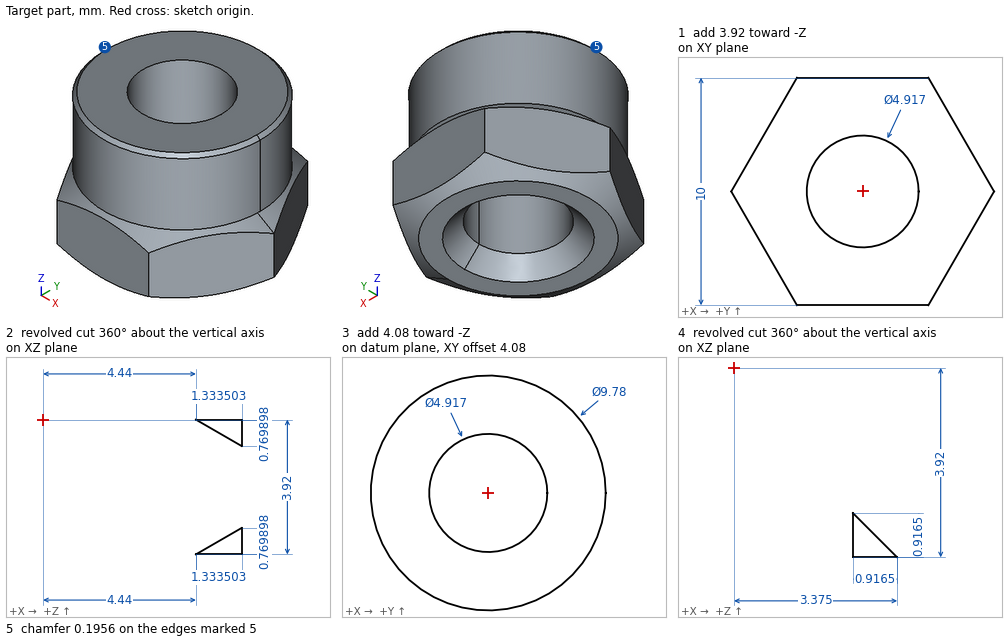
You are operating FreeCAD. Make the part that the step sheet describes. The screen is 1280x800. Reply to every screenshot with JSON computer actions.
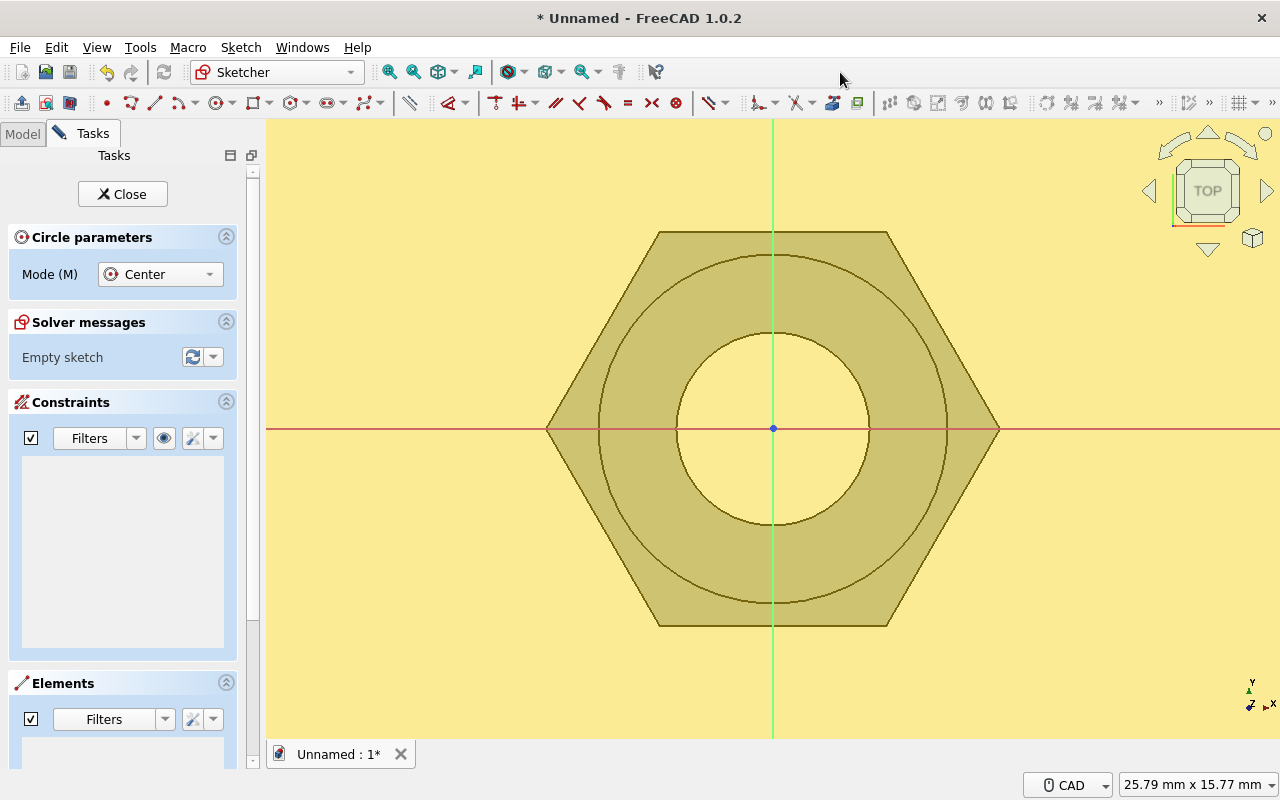
{"action": "left_click", "coordinate": [773, 429]}
{"action": "mouse_move", "coordinate": [909, 293]}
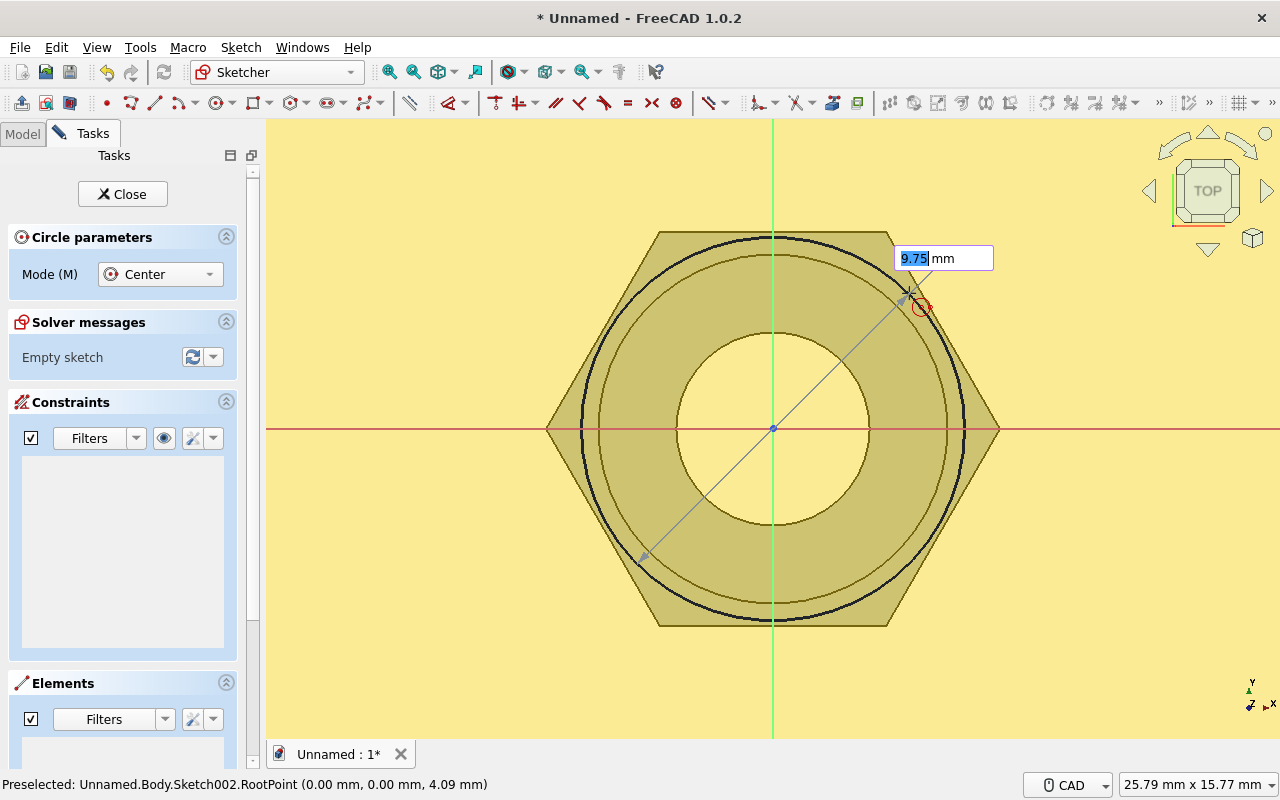
{"action": "type", "text": "9.78"}
{"action": "key", "text": "Return"}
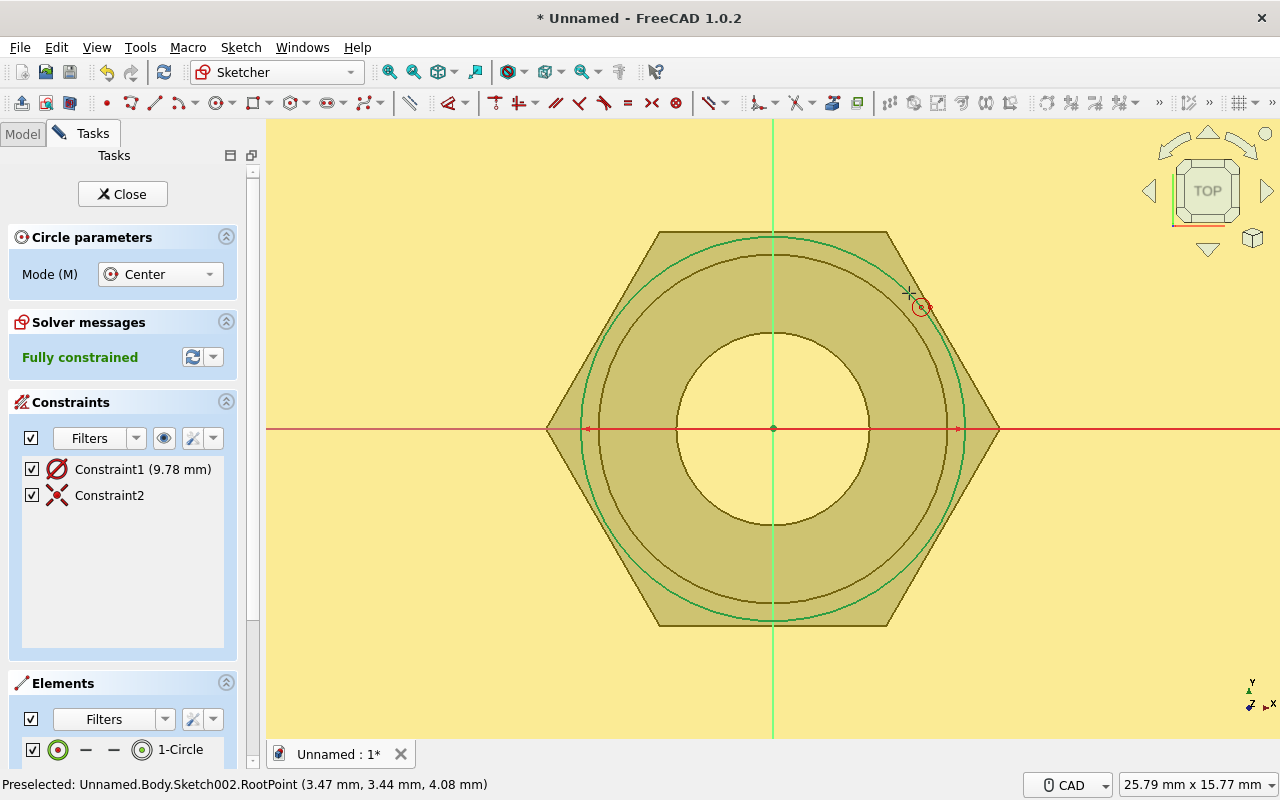
{"action": "left_click", "coordinate": [773, 429]}
{"action": "mouse_move", "coordinate": [841, 361]}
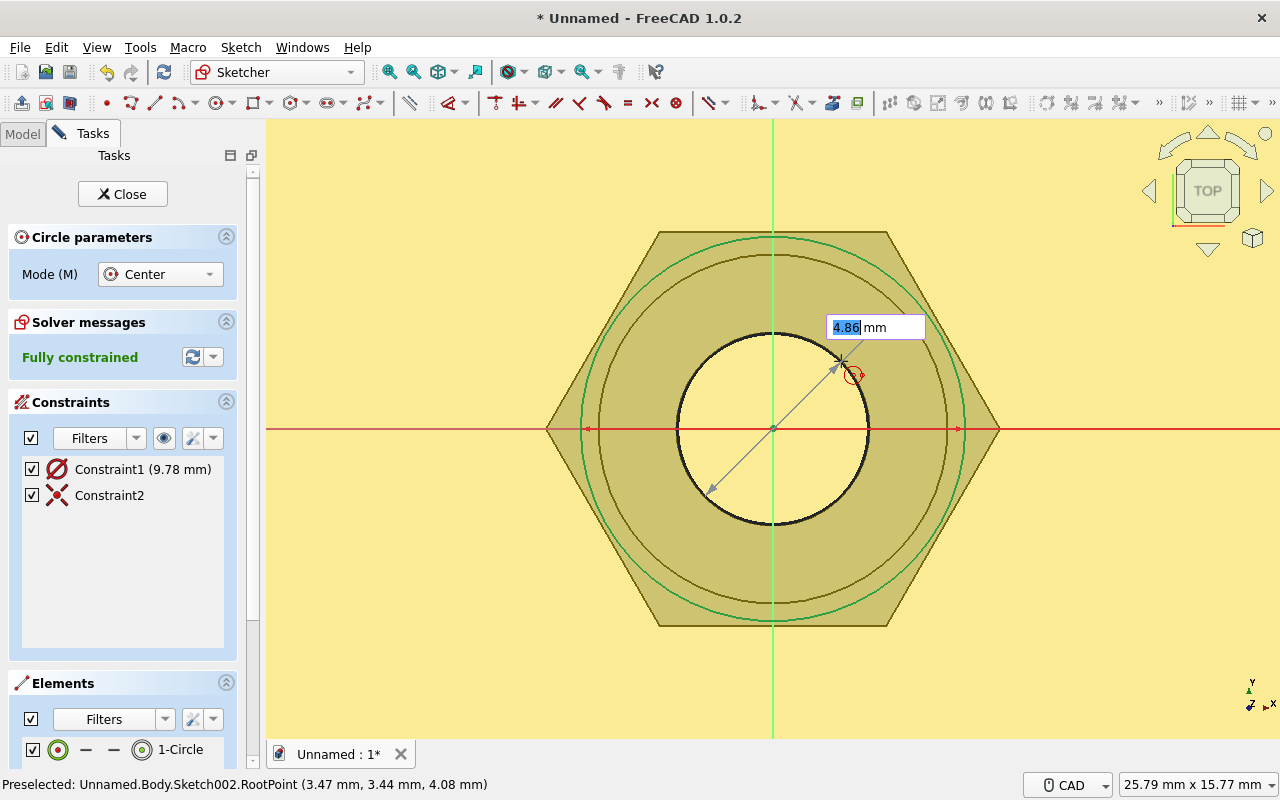
{"action": "type", "text": "4.917"}
{"action": "key", "text": "Return"}
{"action": "key", "text": "Escape"}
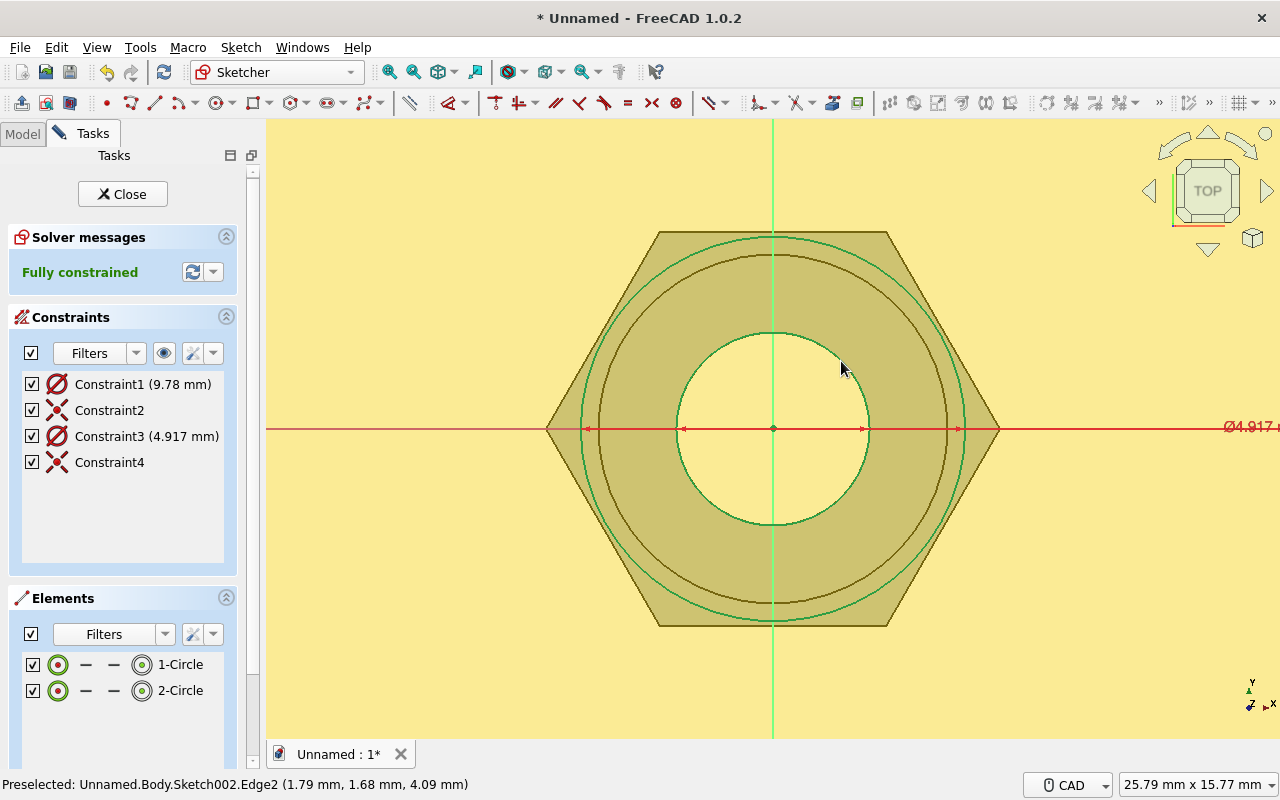
{"action": "left_click", "coordinate": [123, 194]}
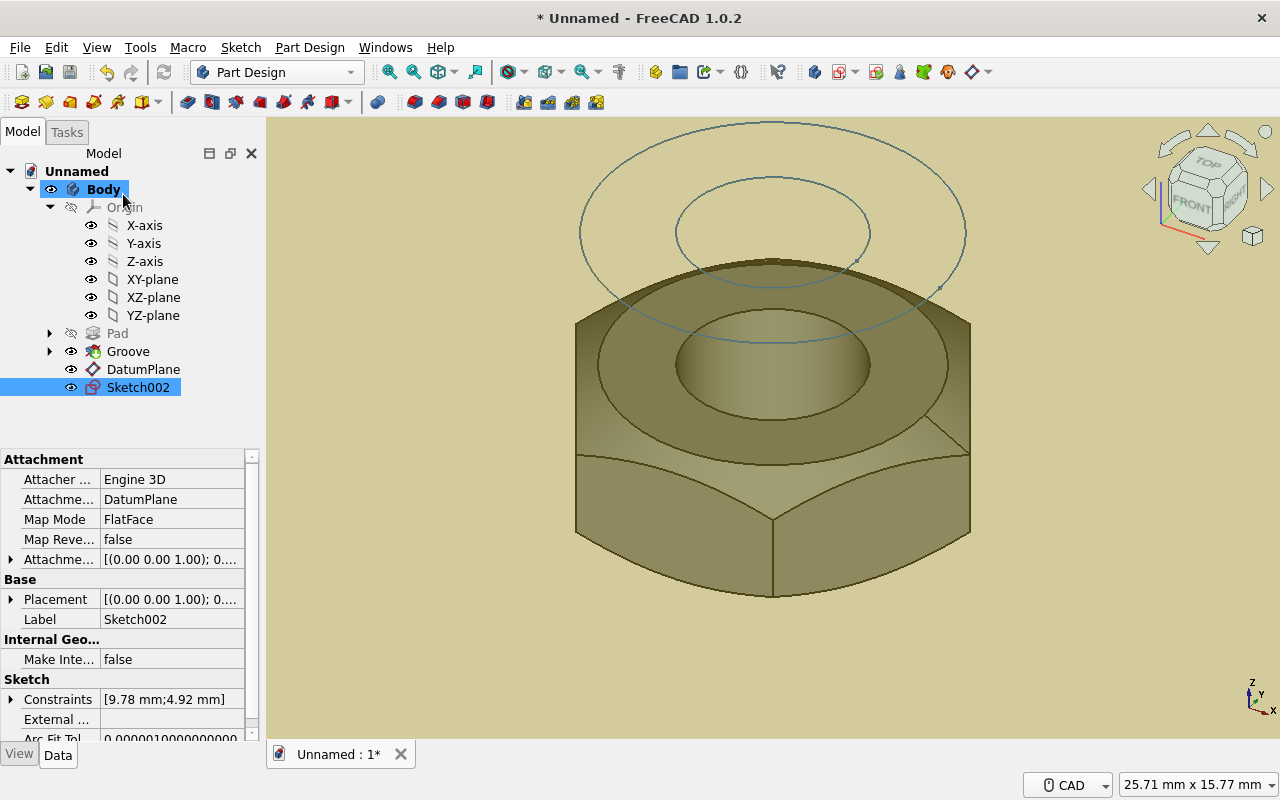
{"action": "left_click", "coordinate": [22, 102]}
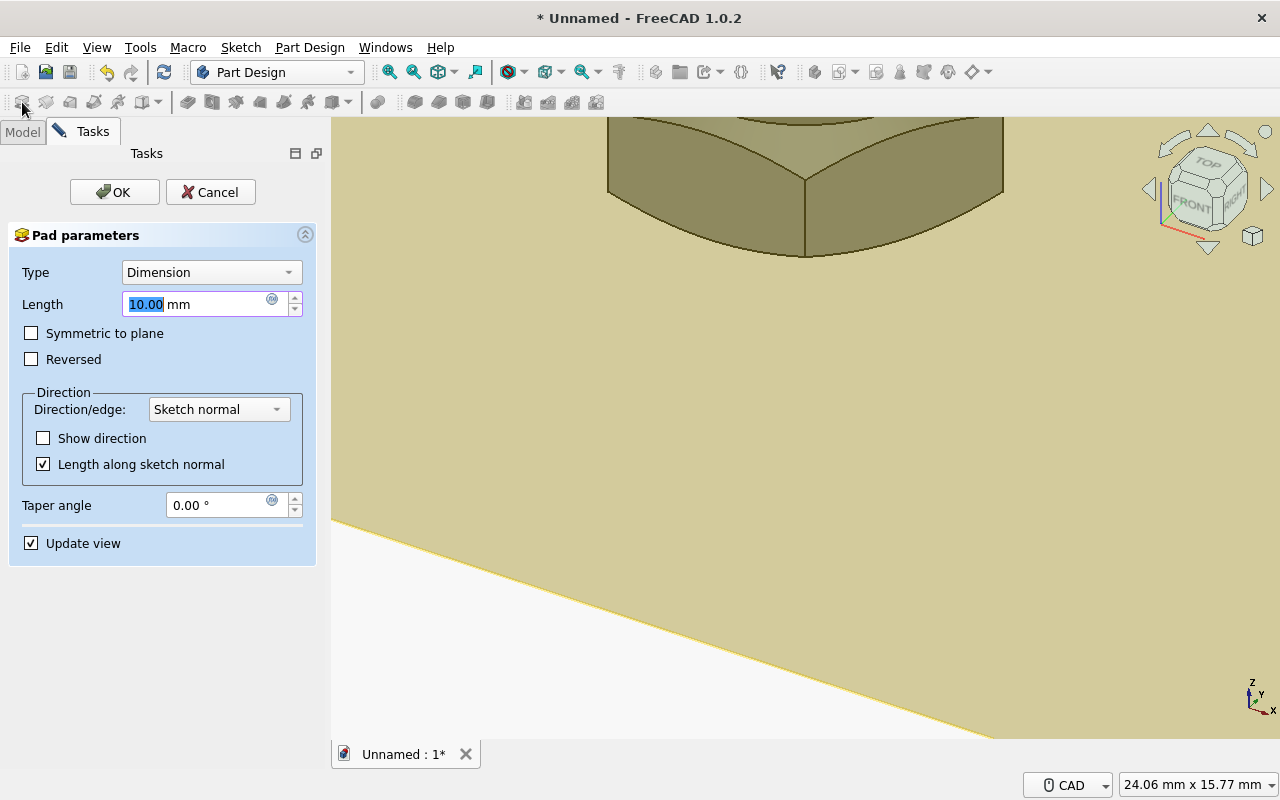
{"action": "type", "text": "4.08"}
{"action": "key", "text": "Tab"}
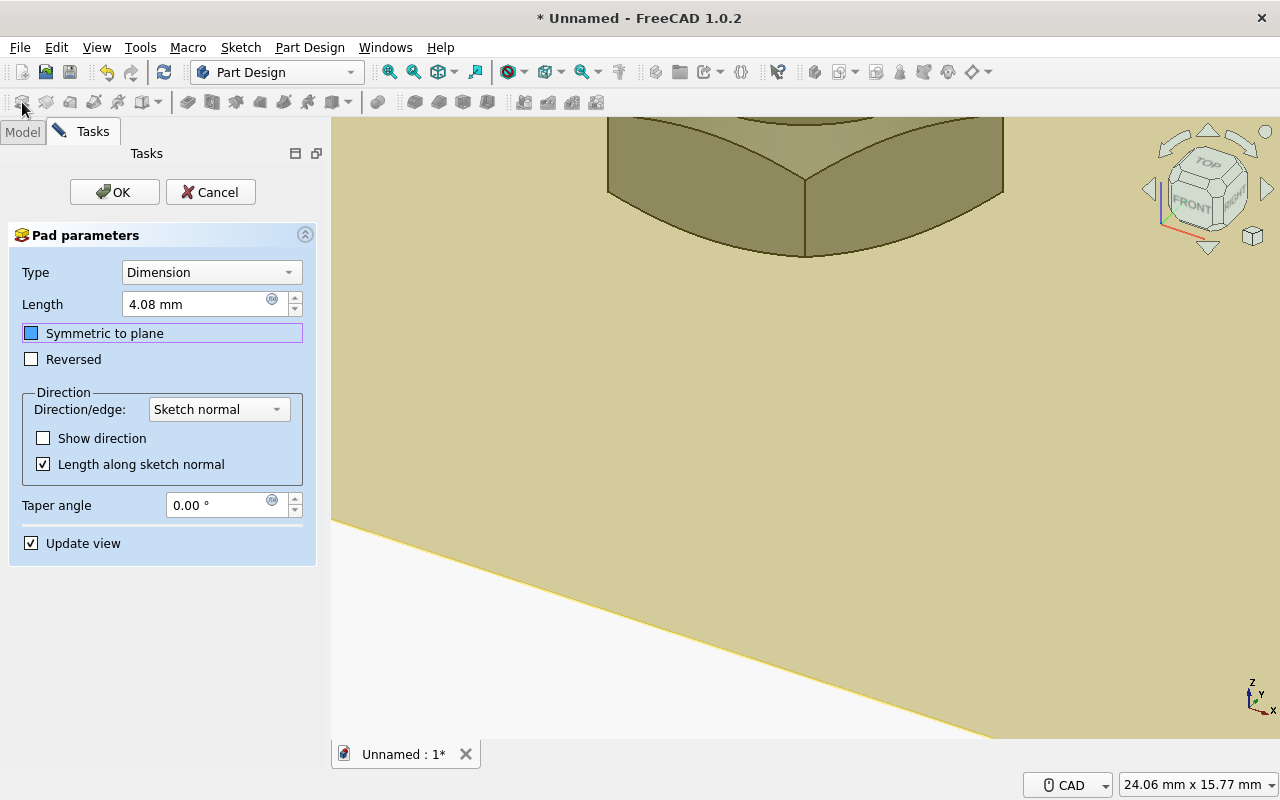
{"action": "left_click", "coordinate": [30, 359]}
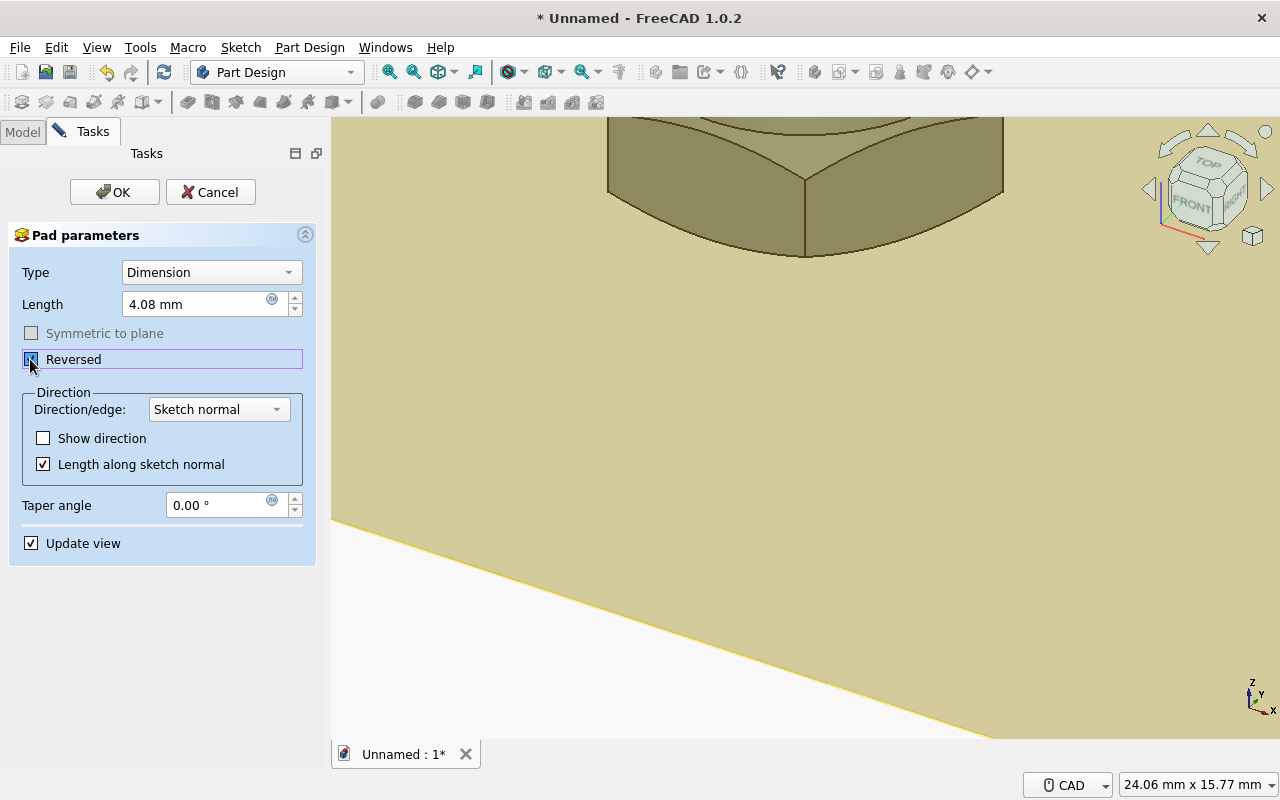
{"action": "left_click", "coordinate": [115, 192]}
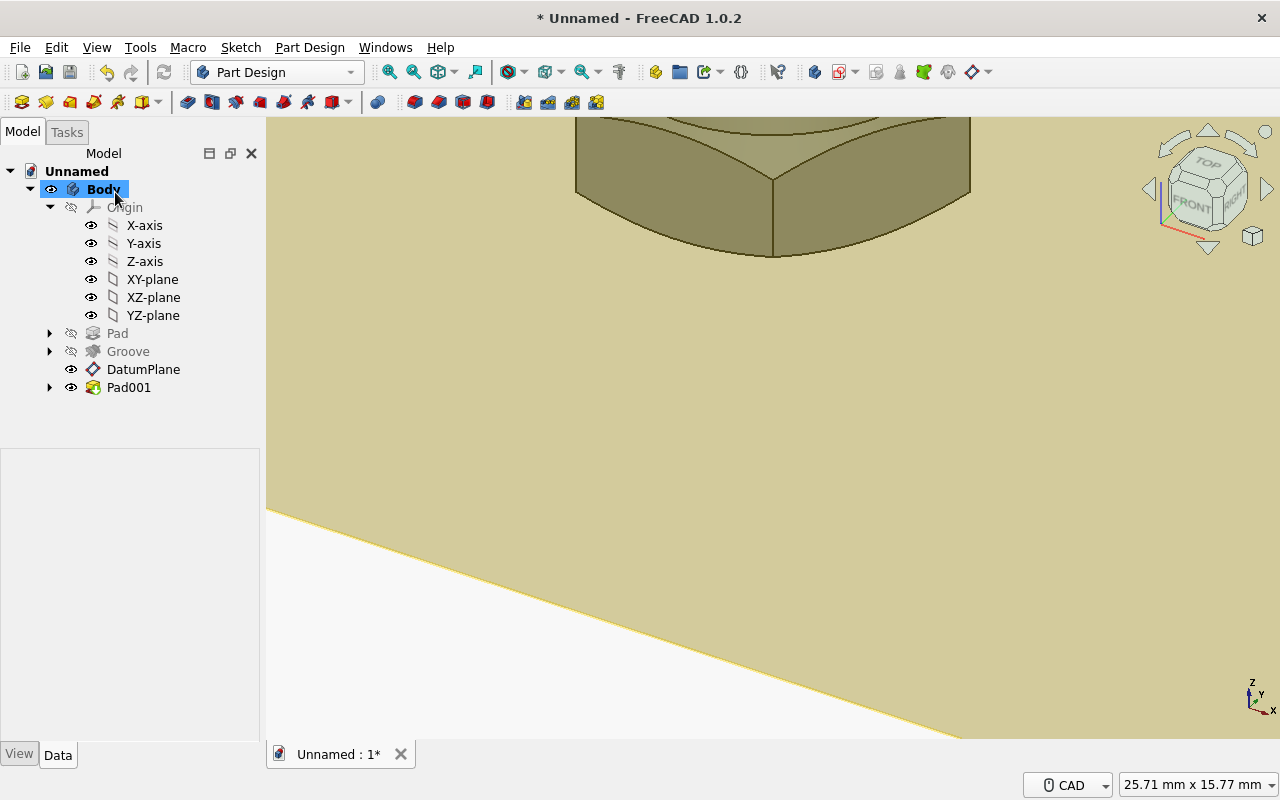
{"action": "left_click", "coordinate": [116, 369]}
{"action": "key", "text": "space"}